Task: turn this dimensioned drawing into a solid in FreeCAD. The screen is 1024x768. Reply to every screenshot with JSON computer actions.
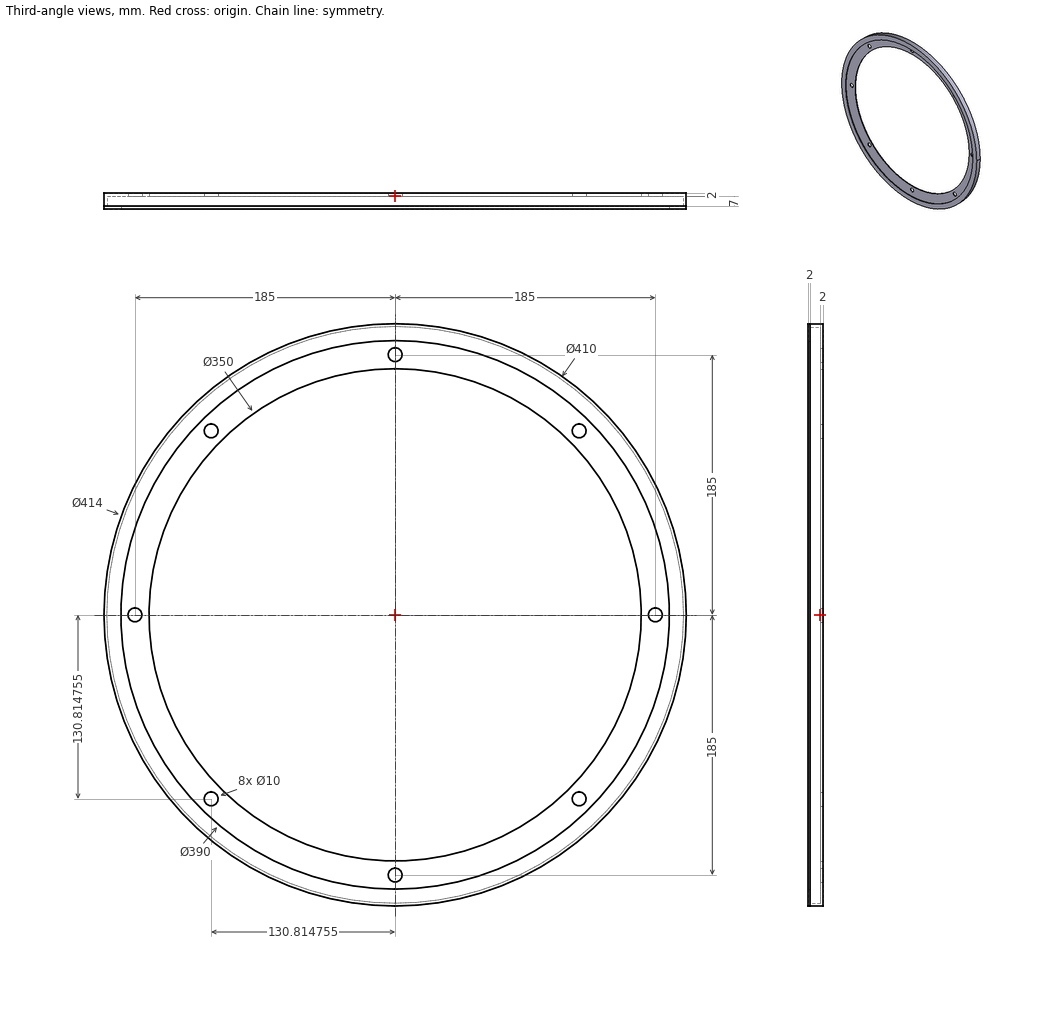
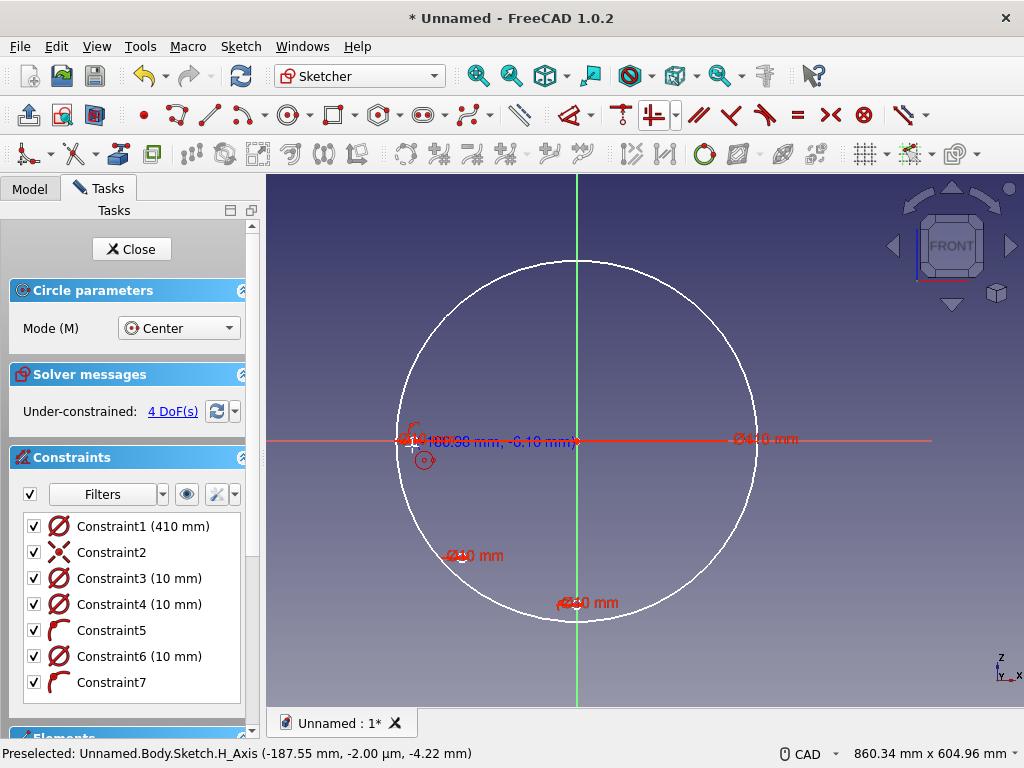
{"action": "scroll", "coordinate": [462, 326], "scroll_direction": "up", "scroll_amount": 9}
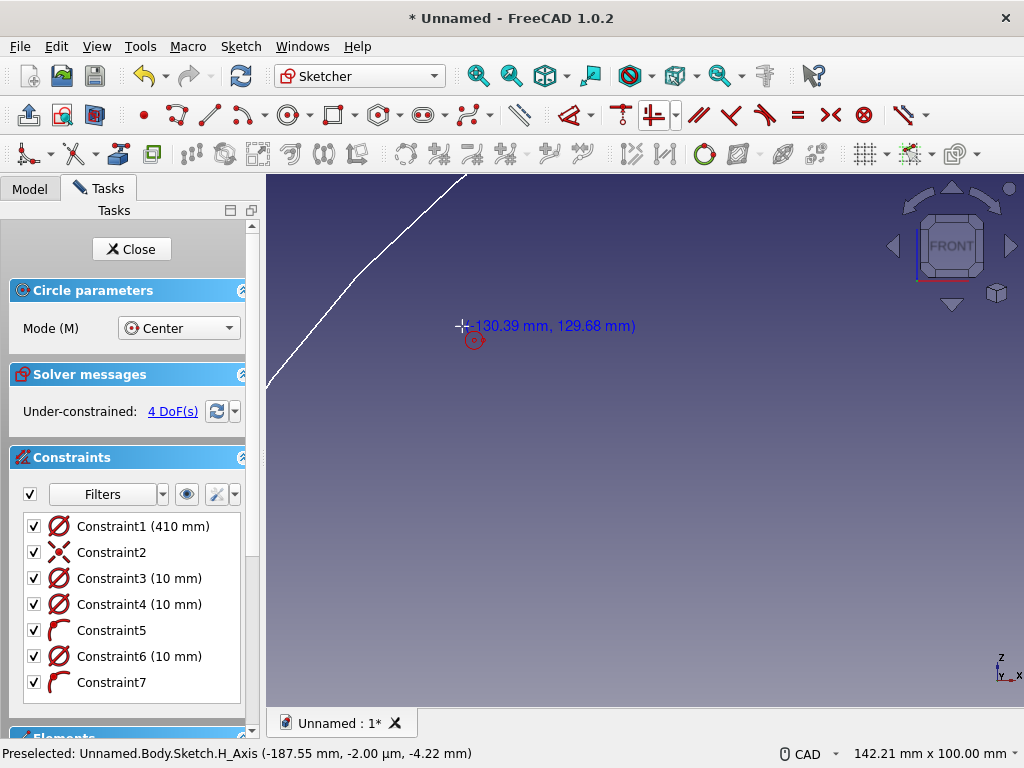
{"action": "scroll", "coordinate": [462, 325], "scroll_direction": "down", "scroll_amount": 9}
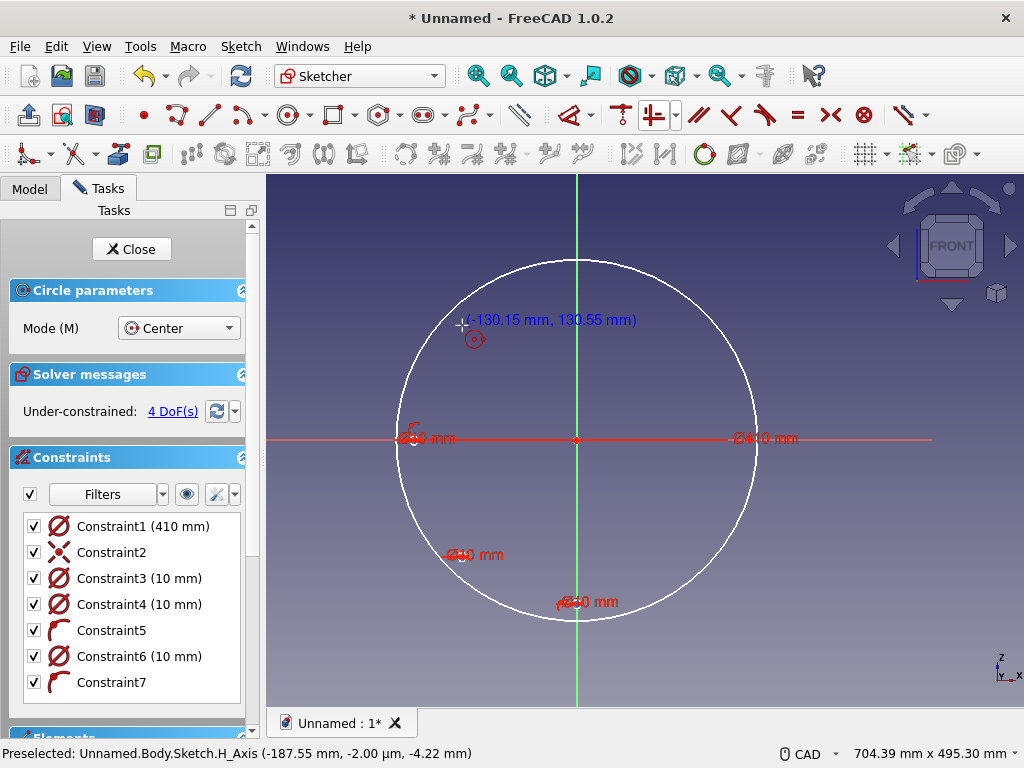
{"action": "left_click", "coordinate": [462, 325]}
{"action": "mouse_move", "coordinate": [465, 322]}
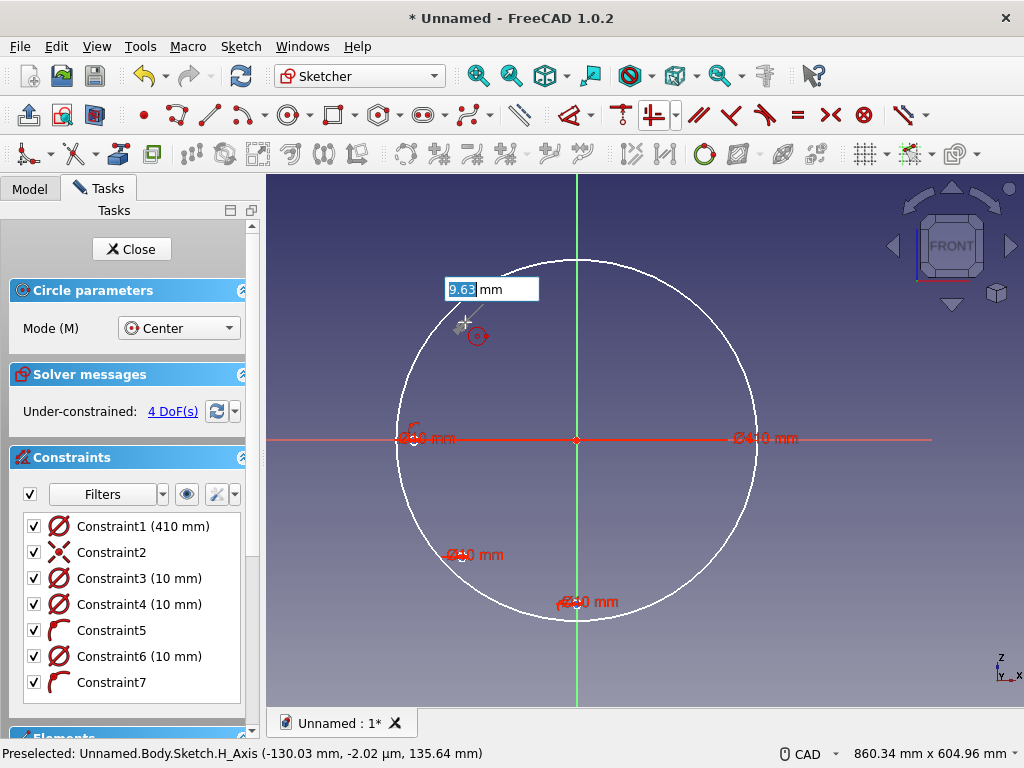
{"action": "type", "text": "10"}
{"action": "key", "text": "Return"}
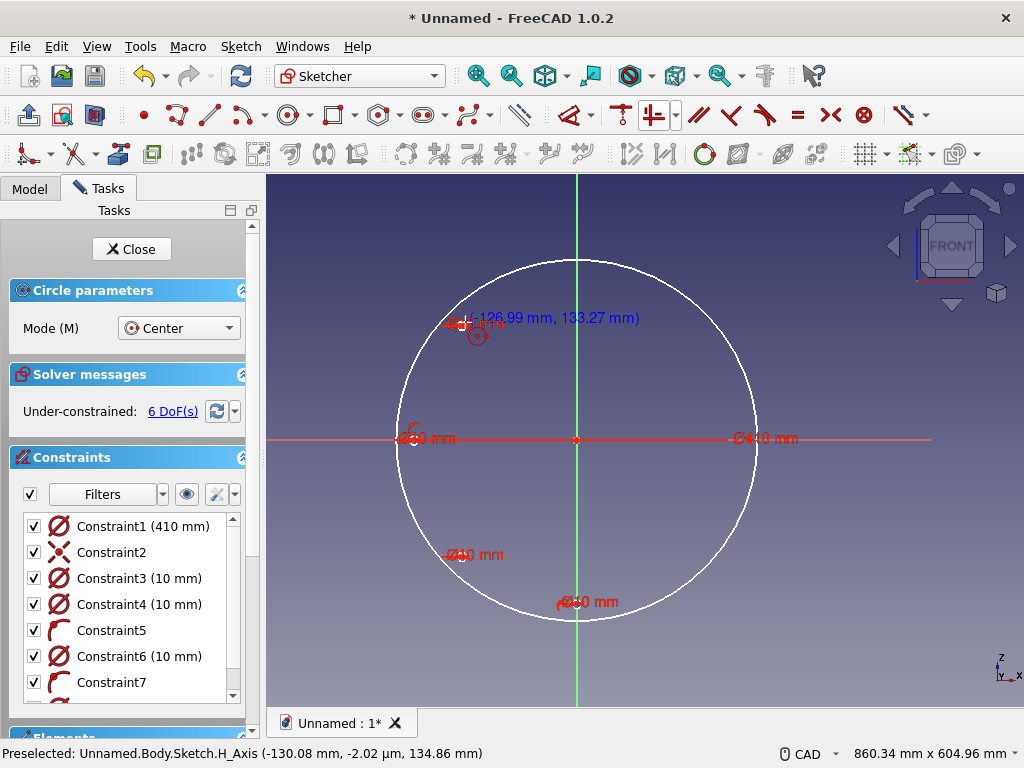
{"action": "scroll", "coordinate": [692, 556], "scroll_direction": "up", "scroll_amount": 9}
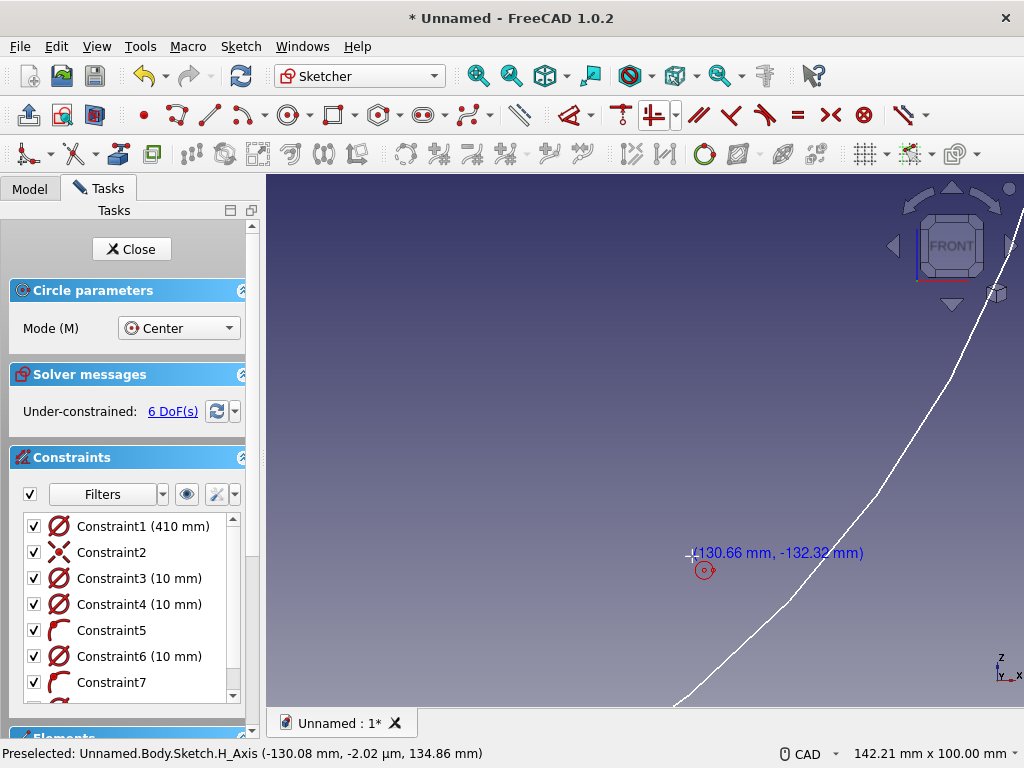
{"action": "scroll", "coordinate": [692, 557], "scroll_direction": "down", "scroll_amount": 9}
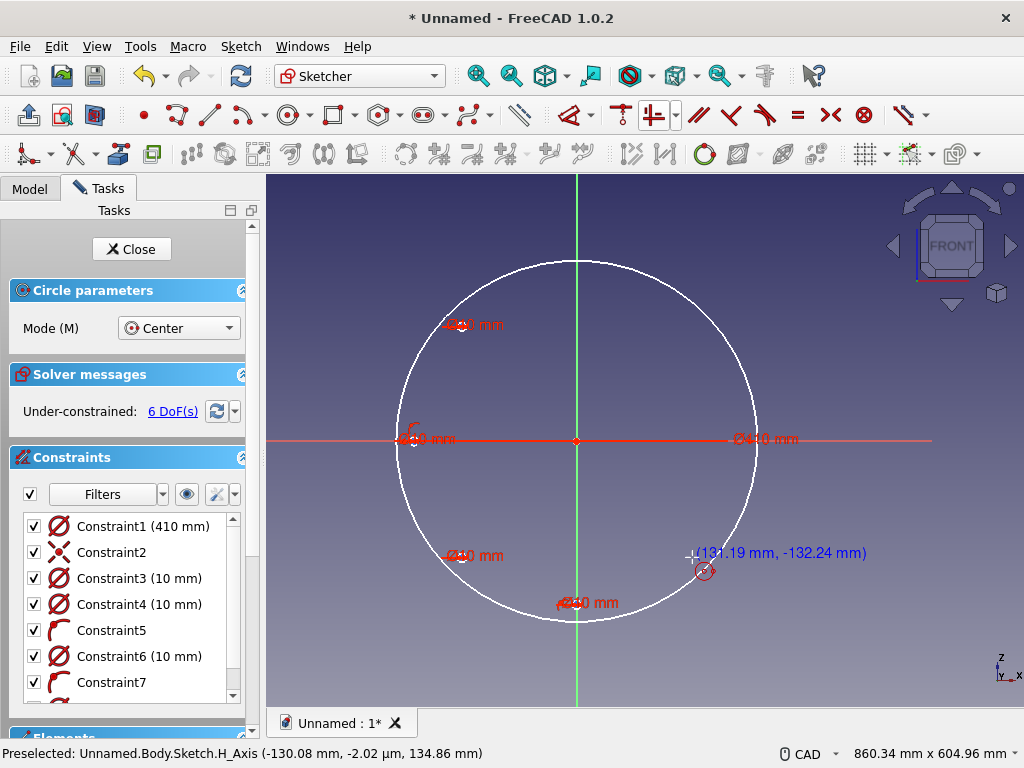
{"action": "left_click", "coordinate": [692, 557]}
{"action": "mouse_move", "coordinate": [695, 553]}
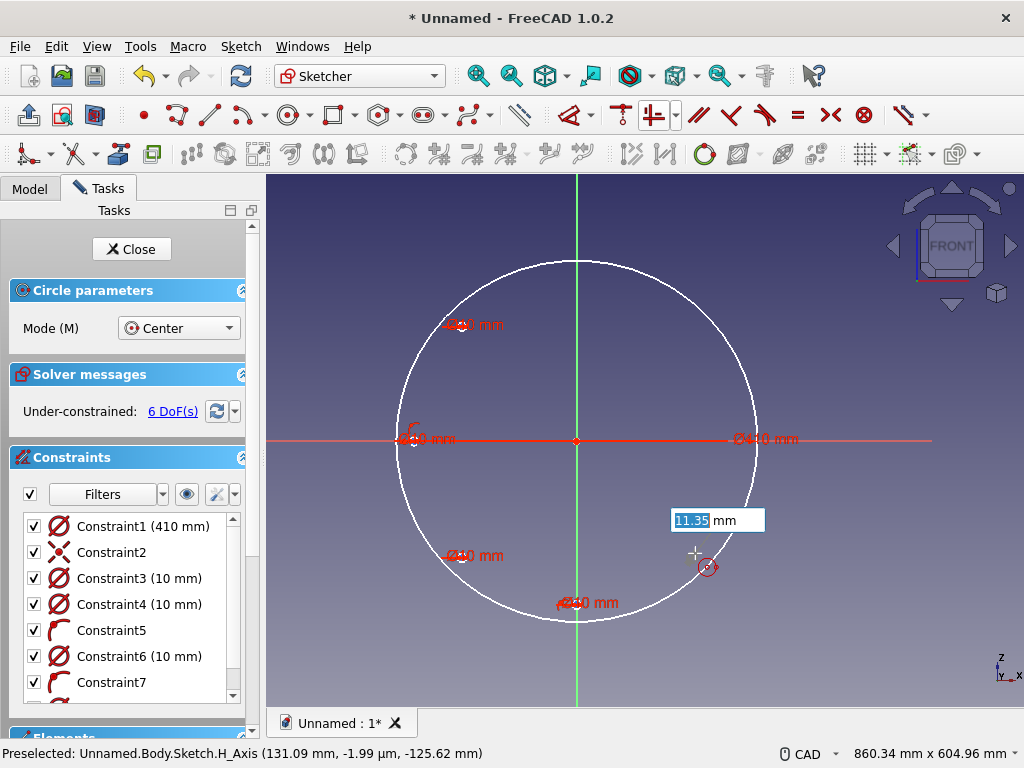
{"action": "type", "text": "10"}
{"action": "key", "text": "Return"}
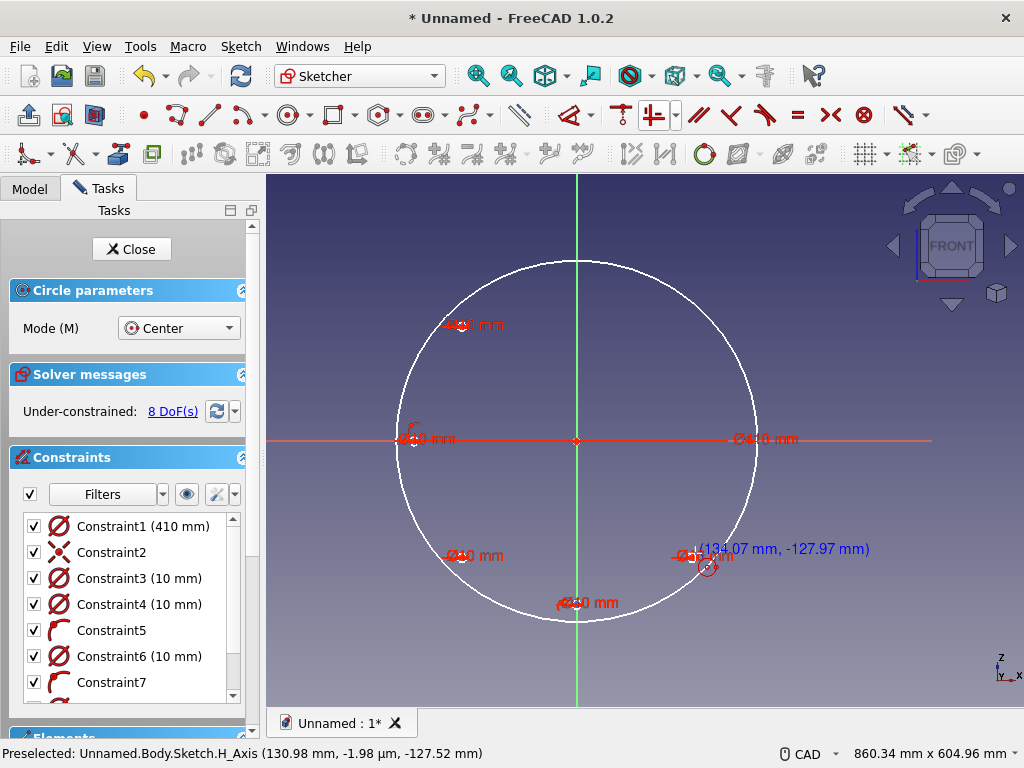
{"action": "scroll", "coordinate": [740, 441], "scroll_direction": "up", "scroll_amount": 9}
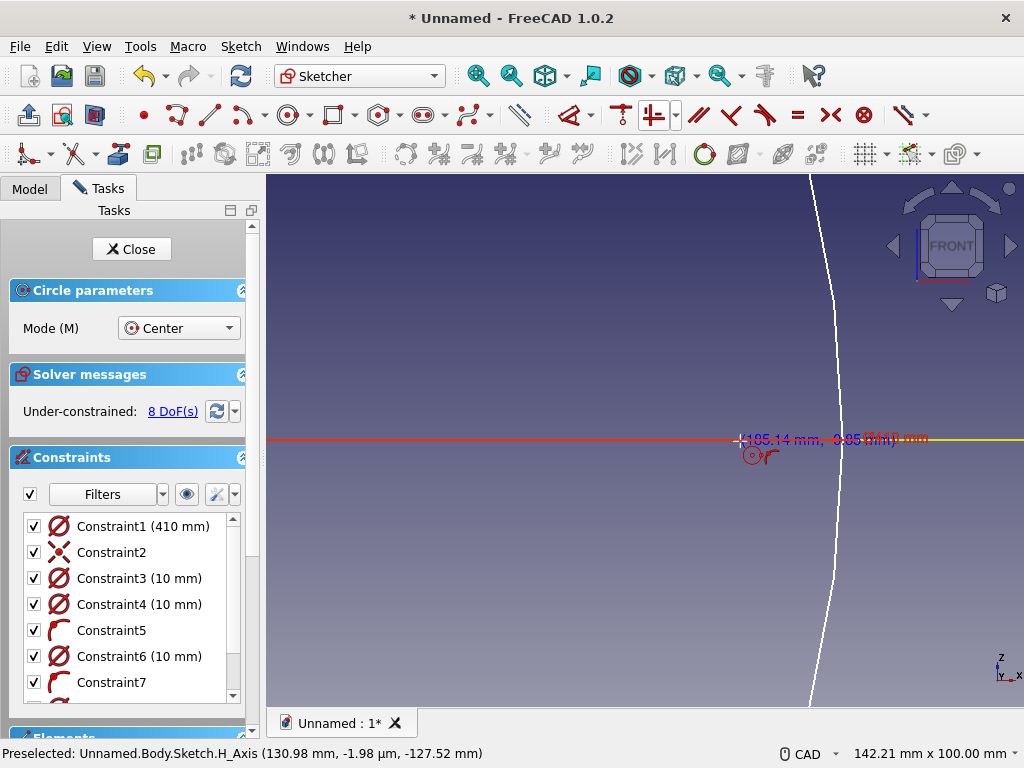
{"action": "scroll", "coordinate": [740, 441], "scroll_direction": "down", "scroll_amount": 9}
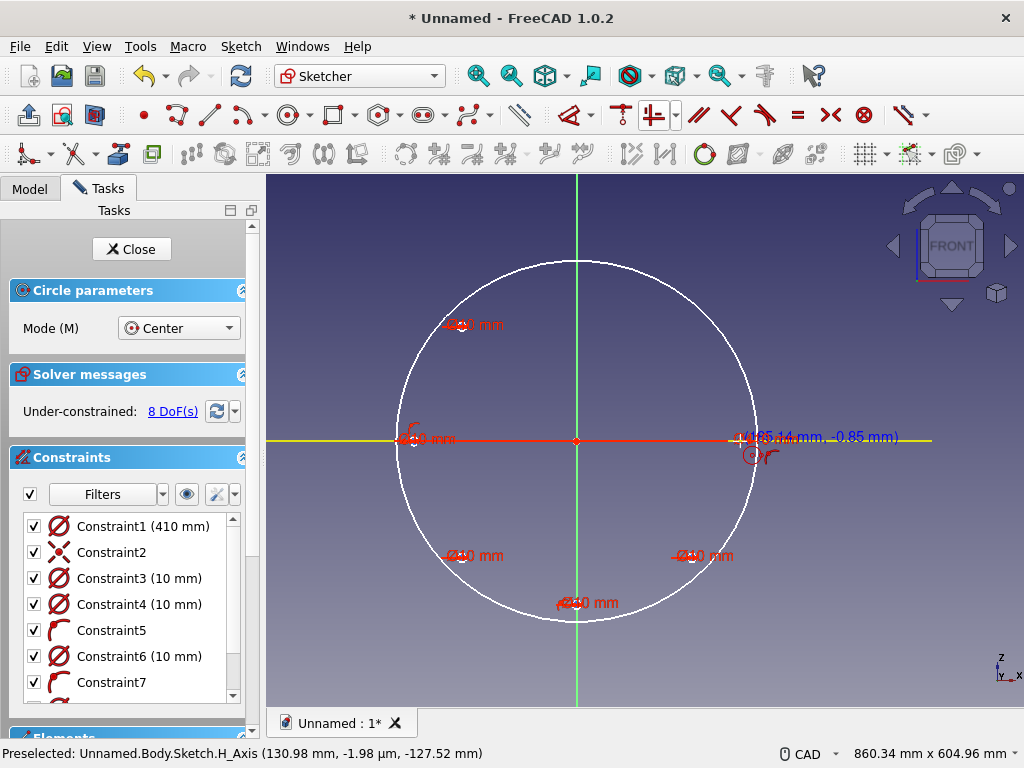
{"action": "left_click", "coordinate": [740, 441]}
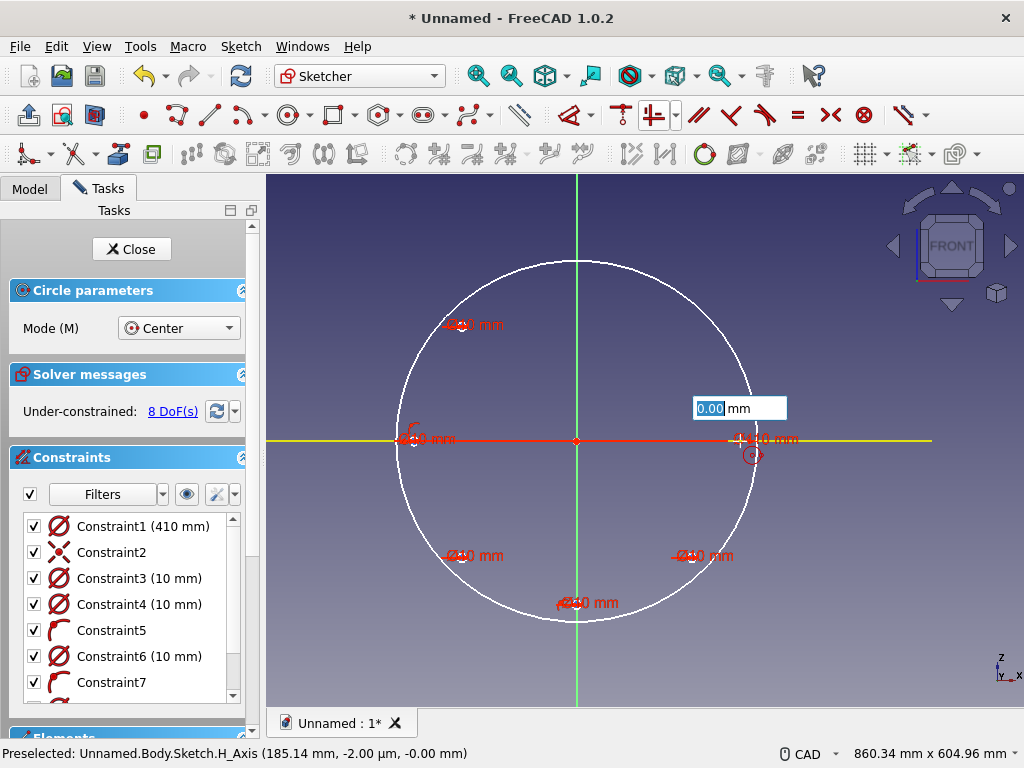
{"action": "scroll", "coordinate": [738, 445], "scroll_direction": "up", "scroll_amount": 7}
{"action": "mouse_move", "coordinate": [738, 445]}